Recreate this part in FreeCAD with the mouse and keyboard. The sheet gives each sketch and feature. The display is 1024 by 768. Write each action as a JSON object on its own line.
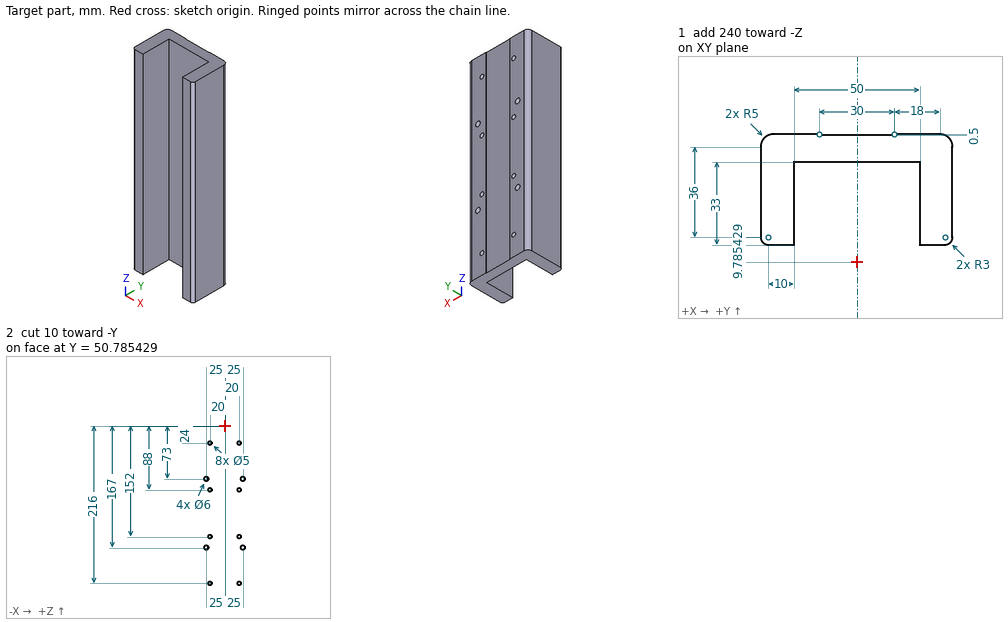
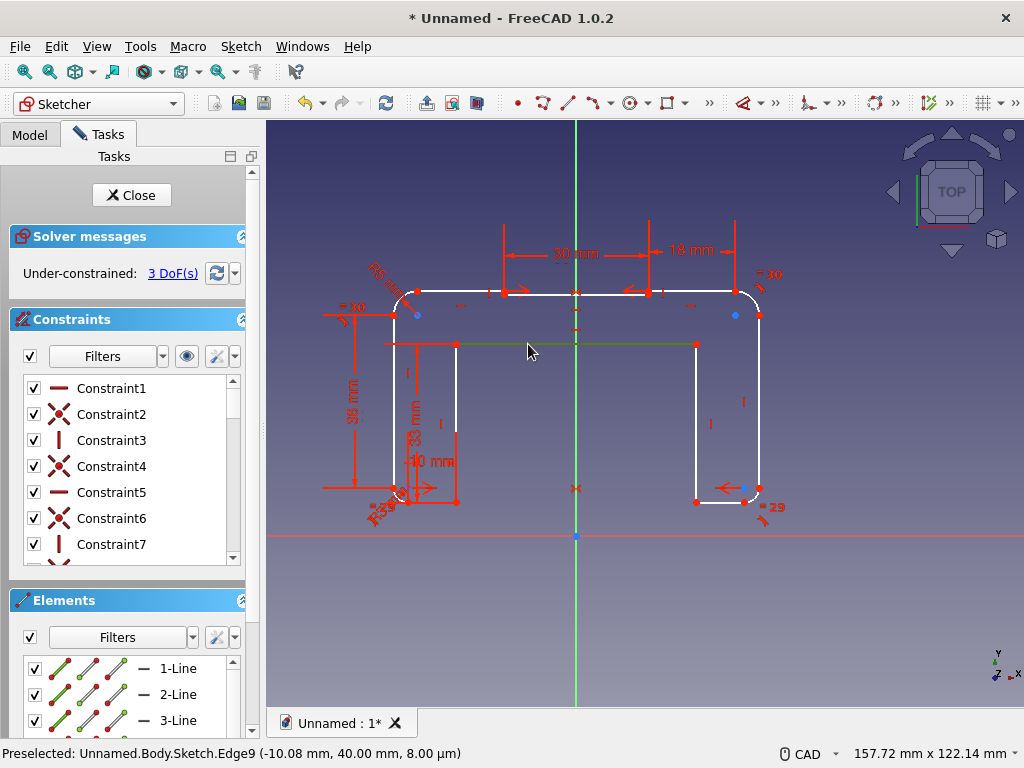
{"action": "left_click", "coordinate": [760, 104]}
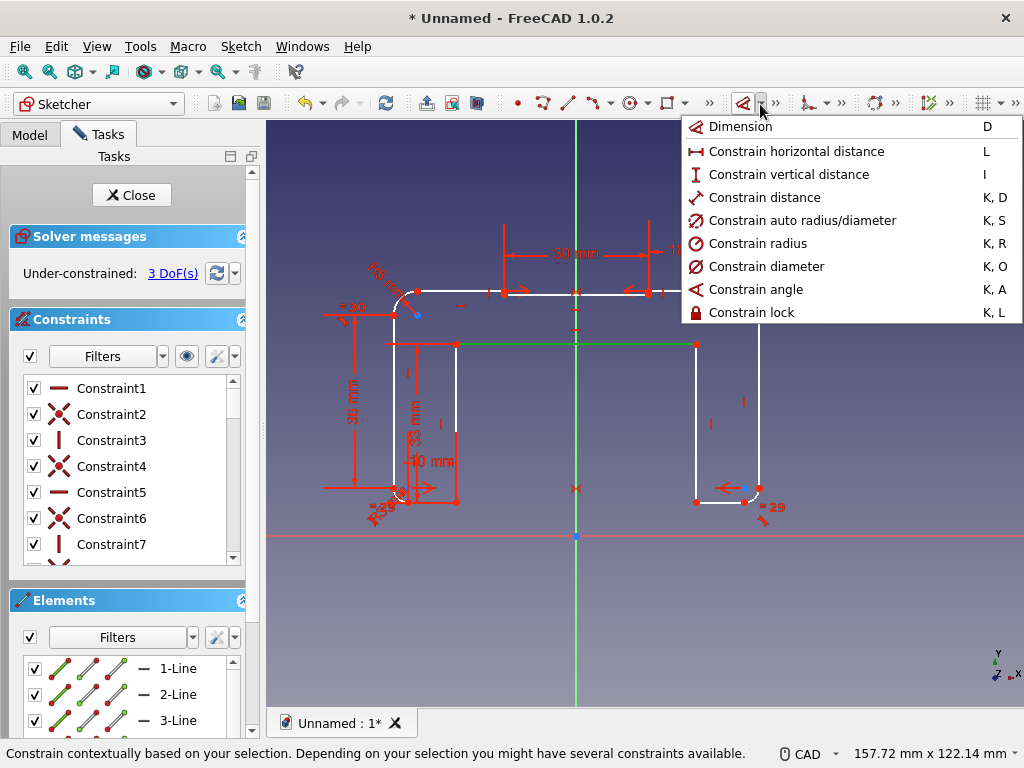
{"action": "left_click", "coordinate": [852, 152]}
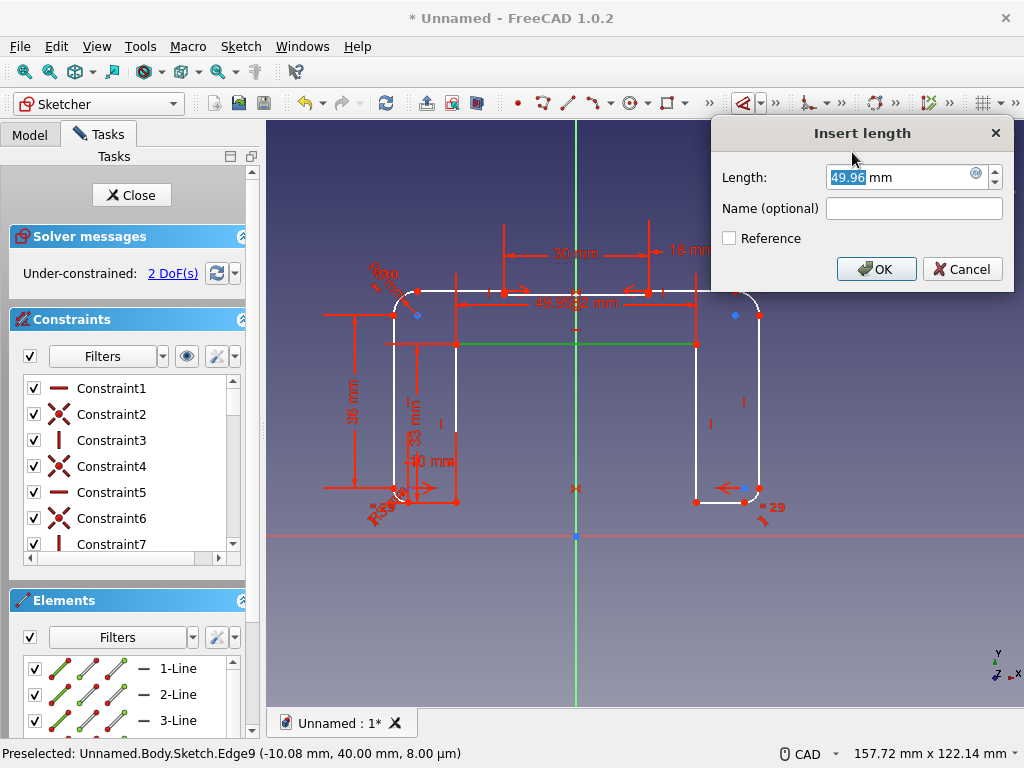
{"action": "type", "text": "50"}
{"action": "key", "text": "Return"}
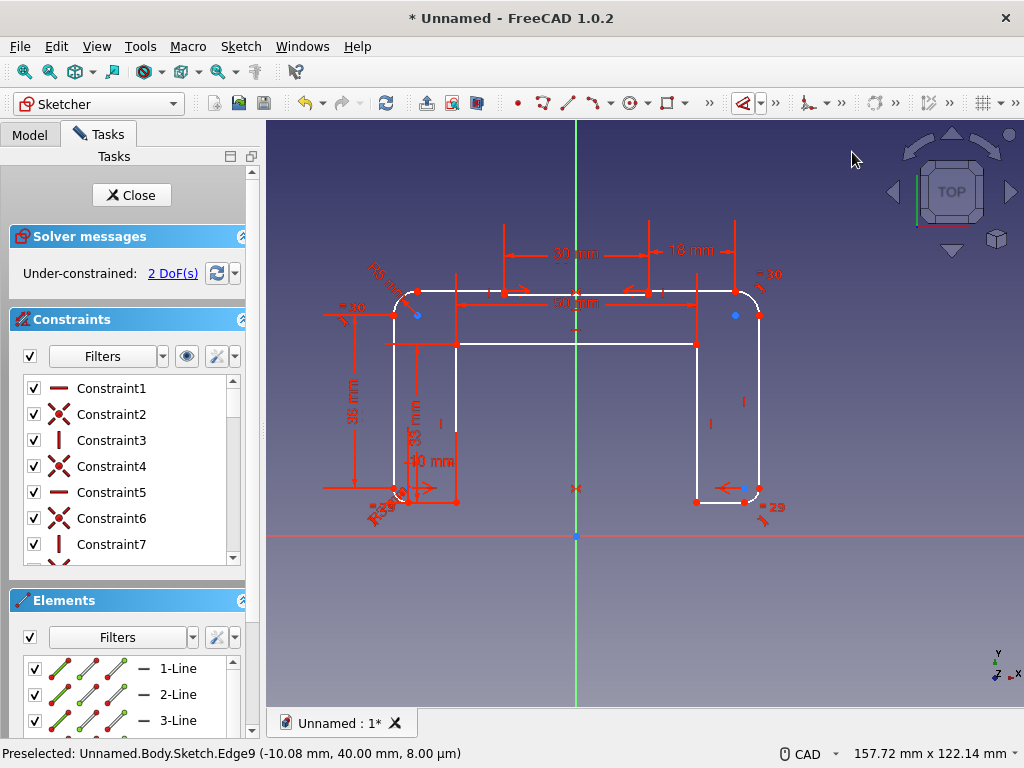
{"action": "scroll", "coordinate": [649, 293], "scroll_direction": "up", "scroll_amount": 15}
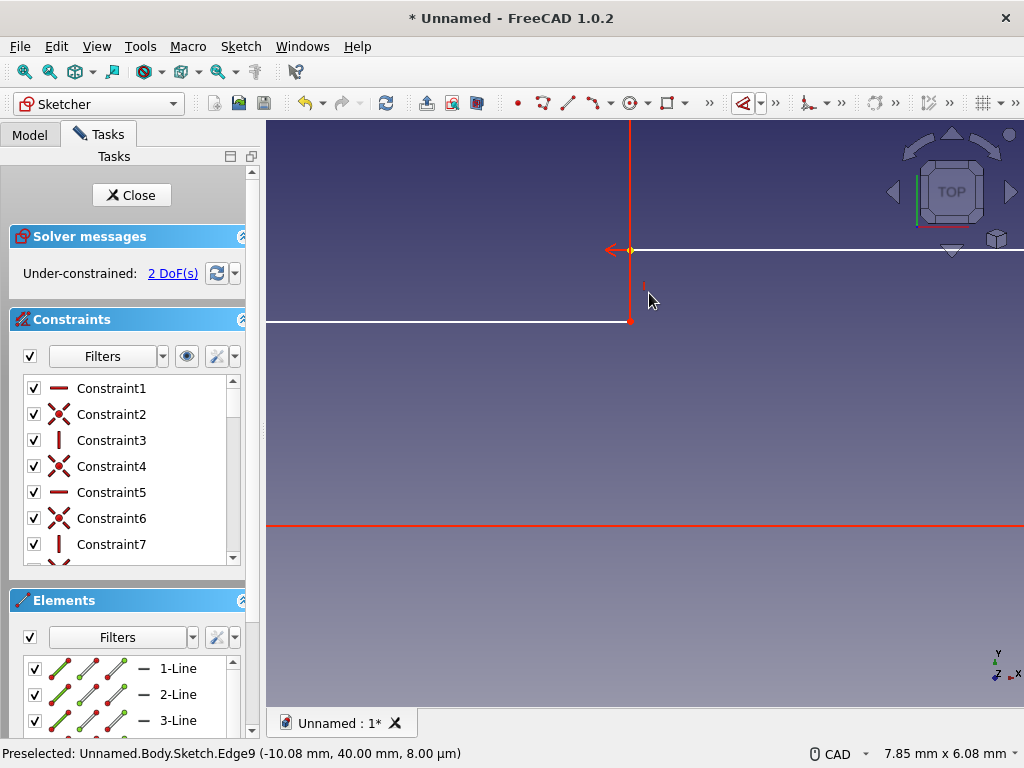
{"action": "left_click", "coordinate": [630, 286]}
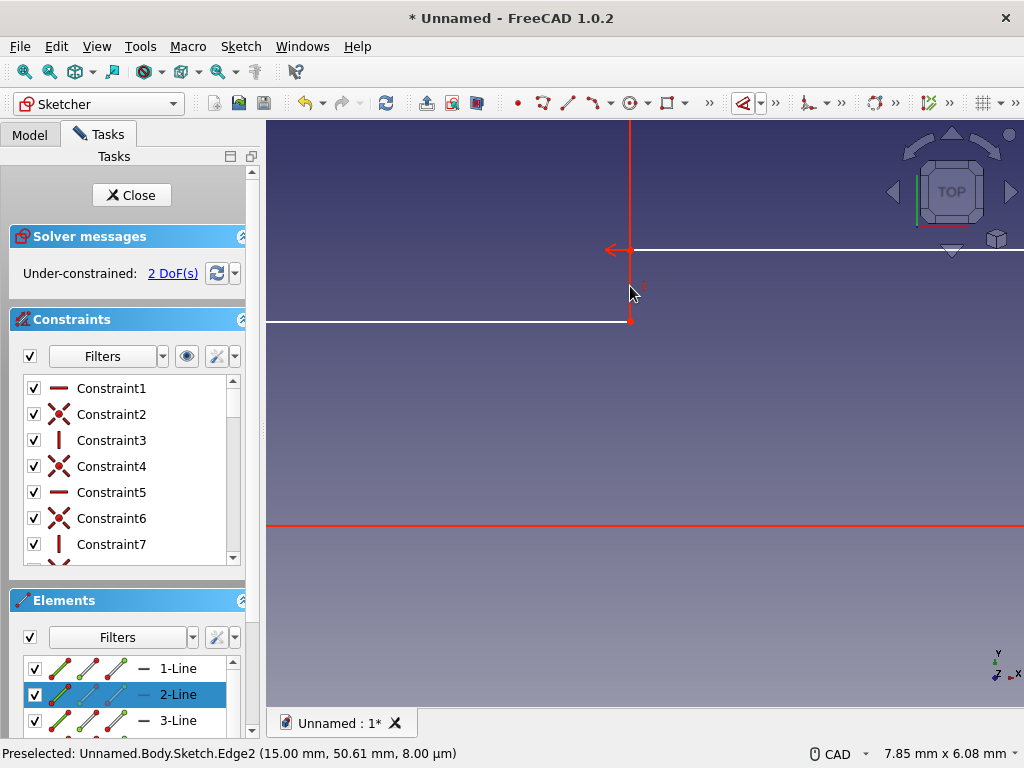
{"action": "key", "text": "i"}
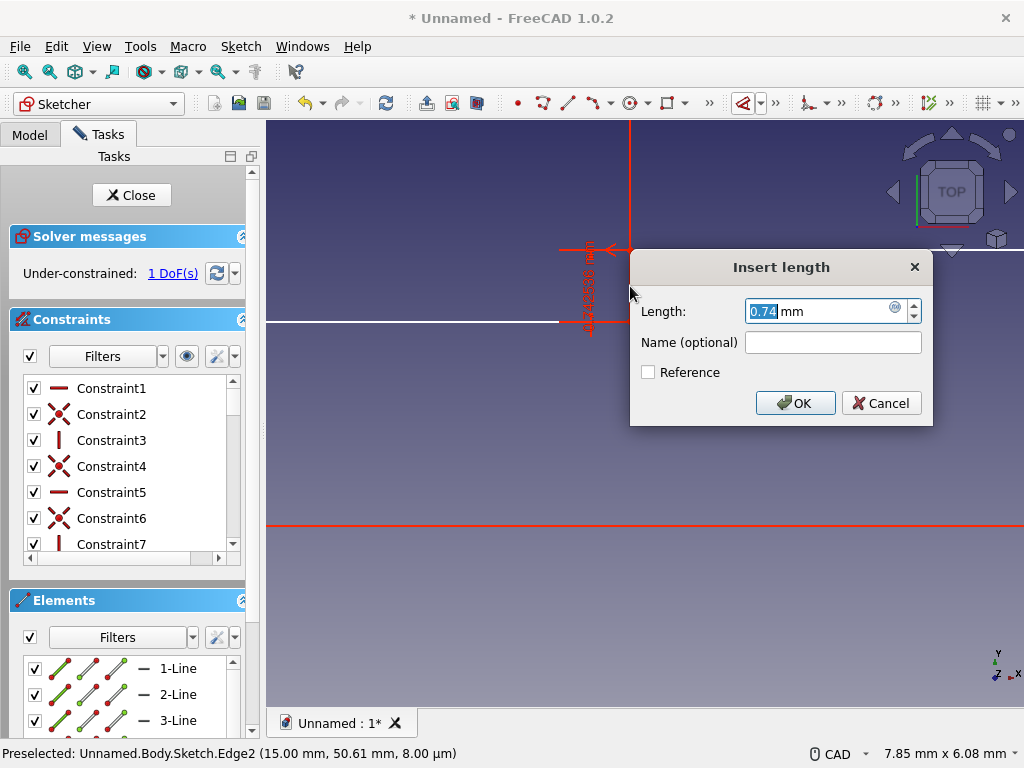
{"action": "type", "text": "0.5"}
{"action": "key", "text": "Return"}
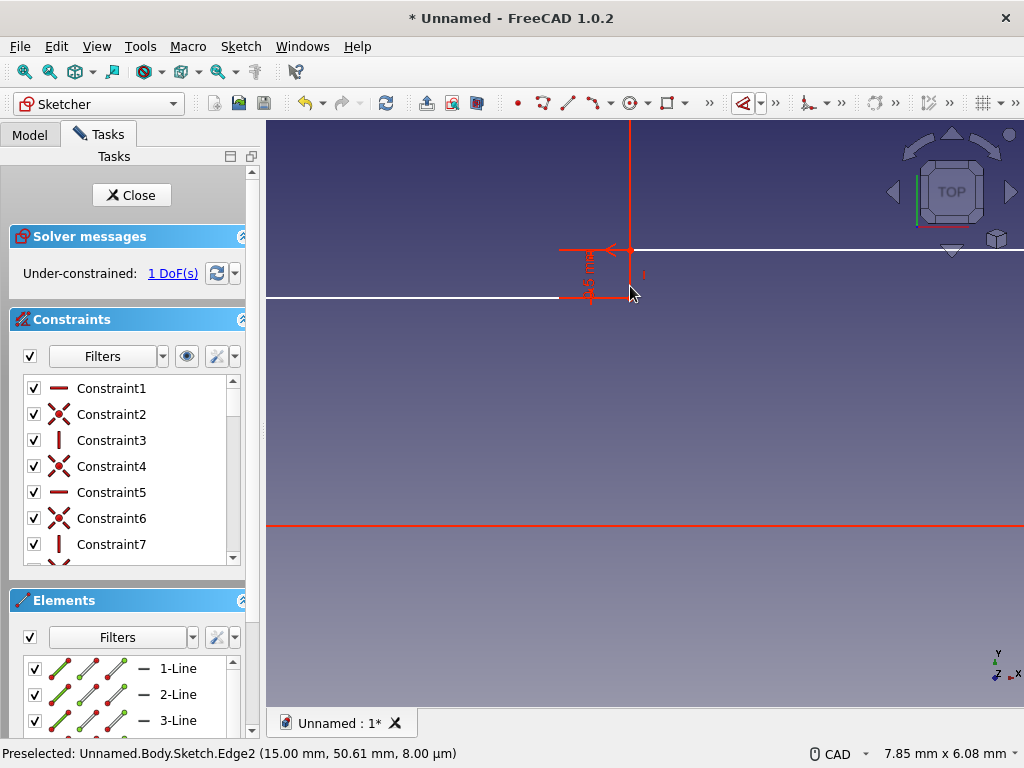
{"action": "scroll", "coordinate": [650, 293], "scroll_direction": "down", "scroll_amount": 15}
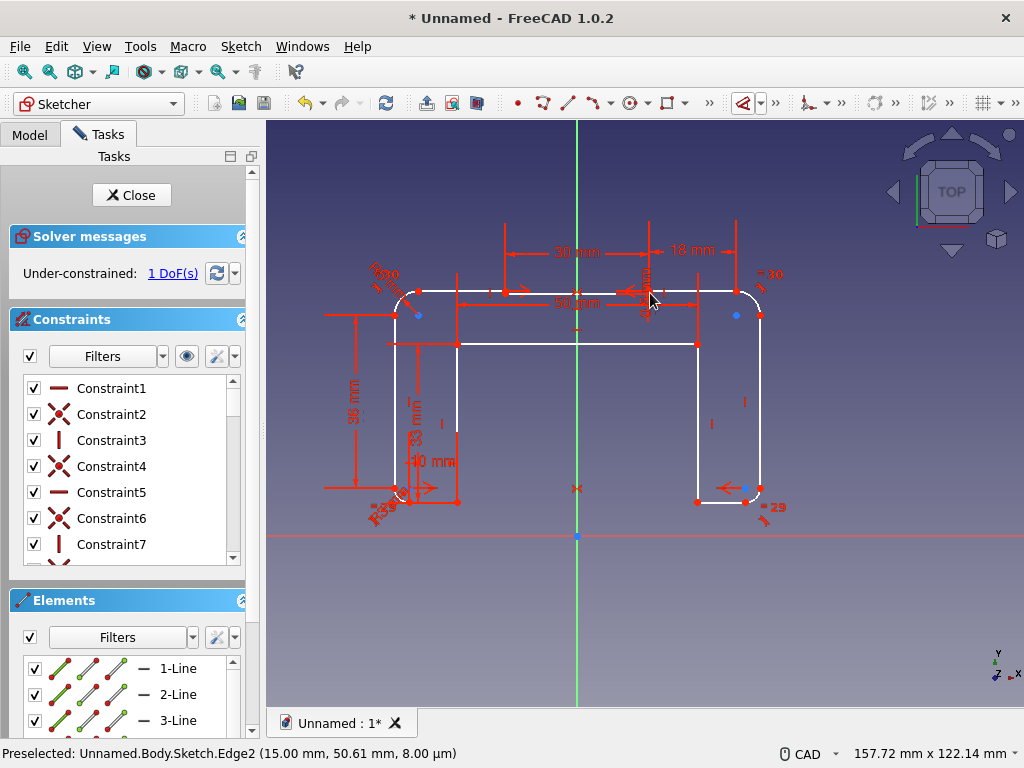
{"action": "left_click", "coordinate": [395, 488]}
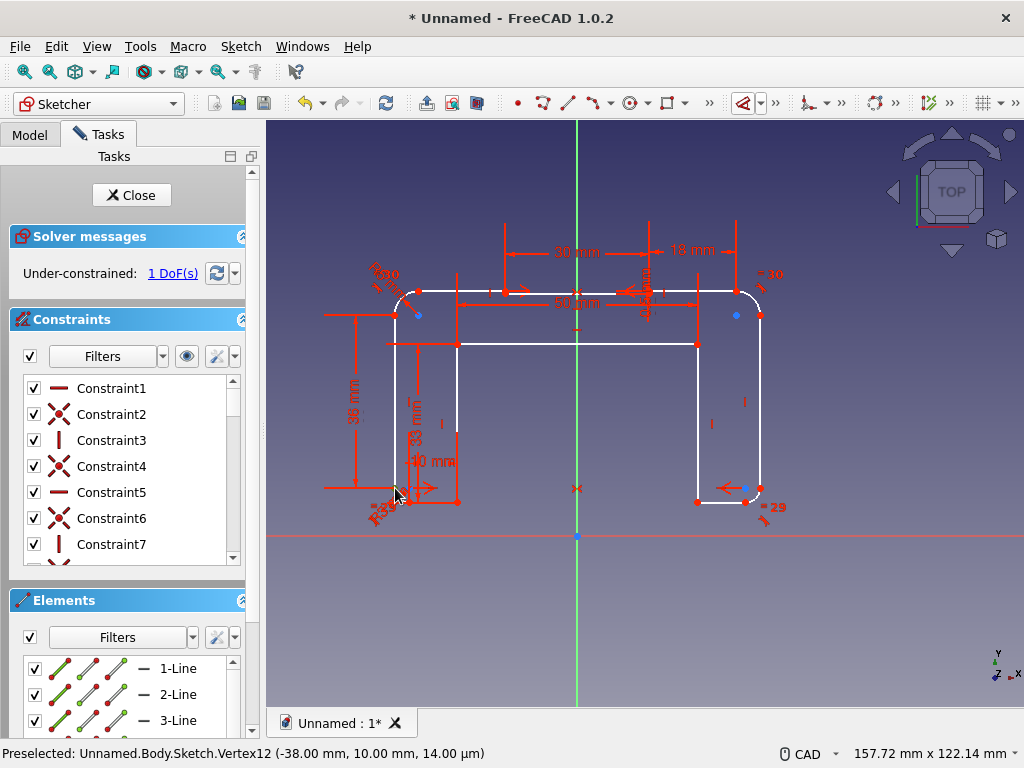
{"action": "key", "text": "i"}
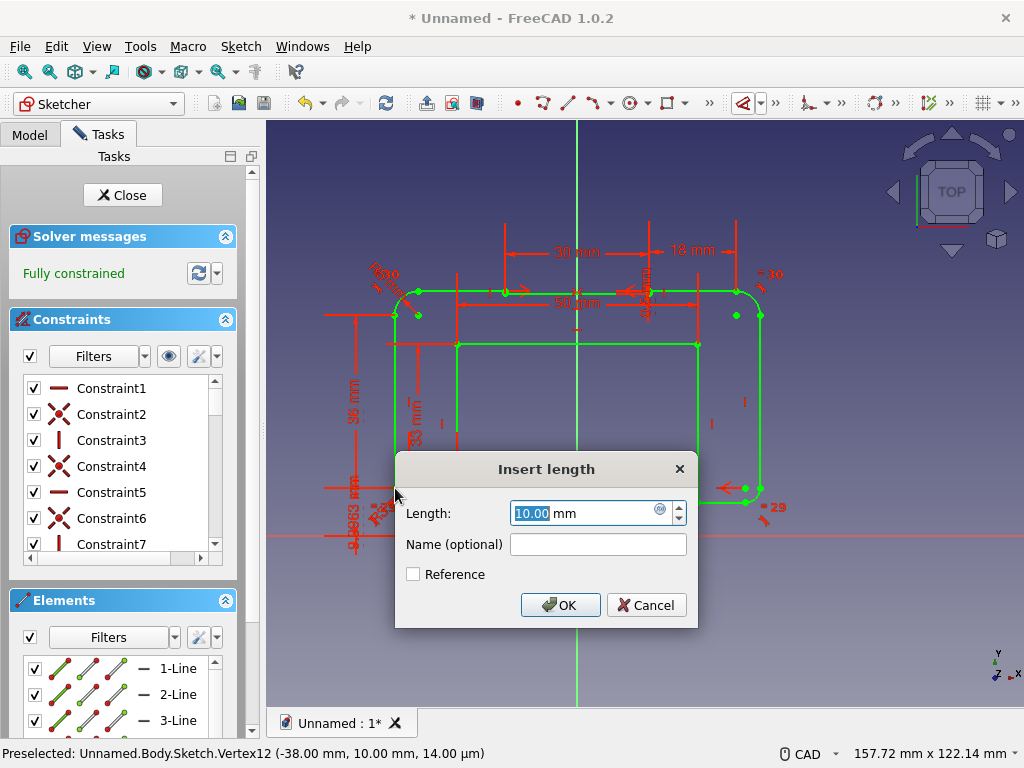
{"action": "type", "text": "9.785429"}
{"action": "key", "text": "Return"}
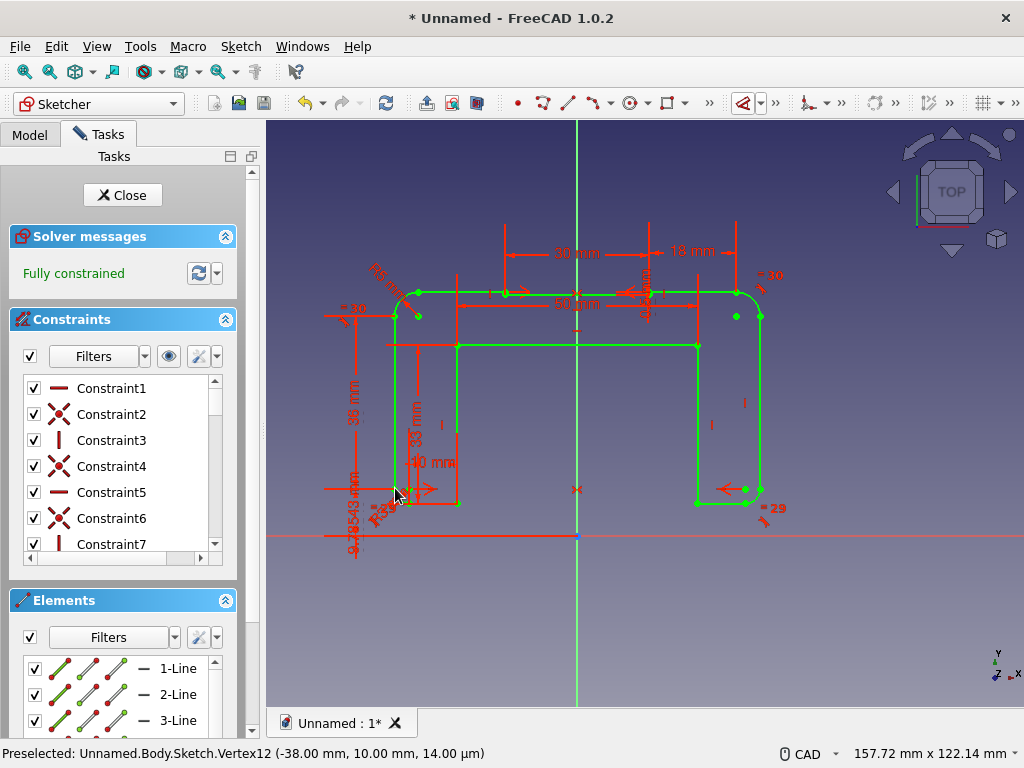
{"action": "left_click", "coordinate": [123, 195]}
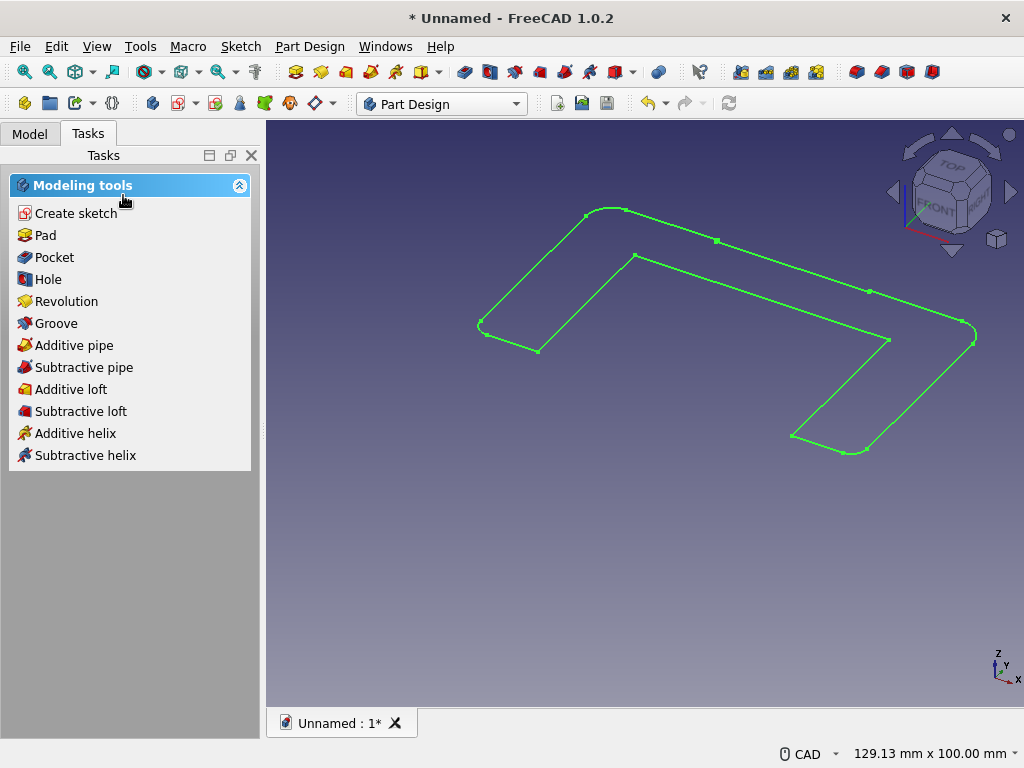
{"action": "left_click", "coordinate": [296, 72]}